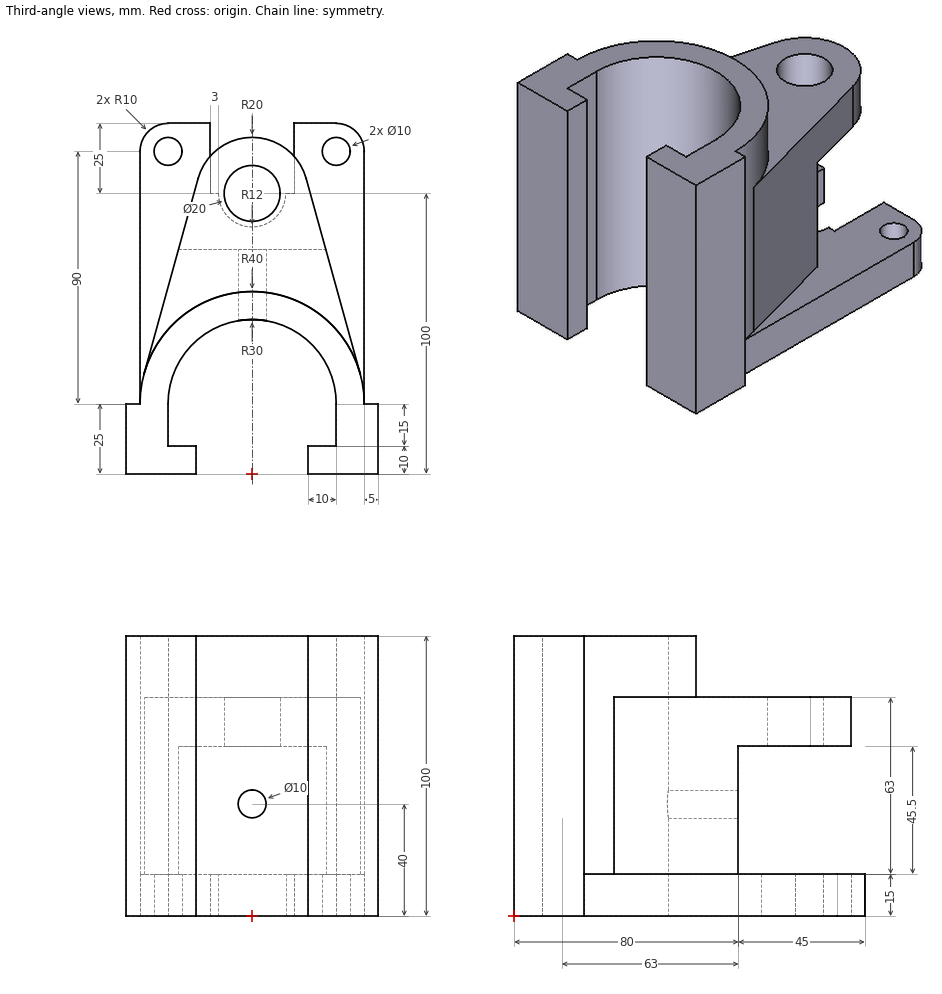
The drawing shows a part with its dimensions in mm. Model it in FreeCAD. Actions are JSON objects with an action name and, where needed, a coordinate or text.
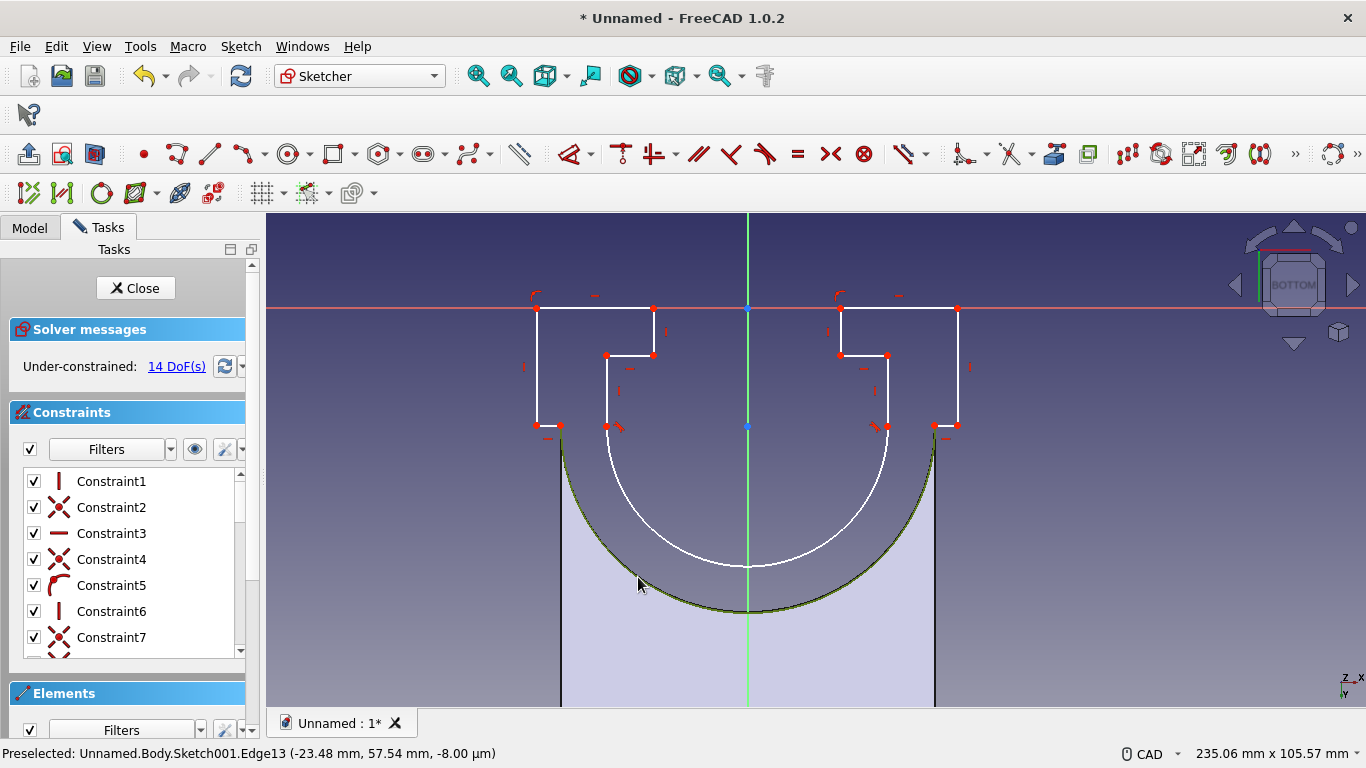
{"action": "left_click", "coordinate": [665, 540]}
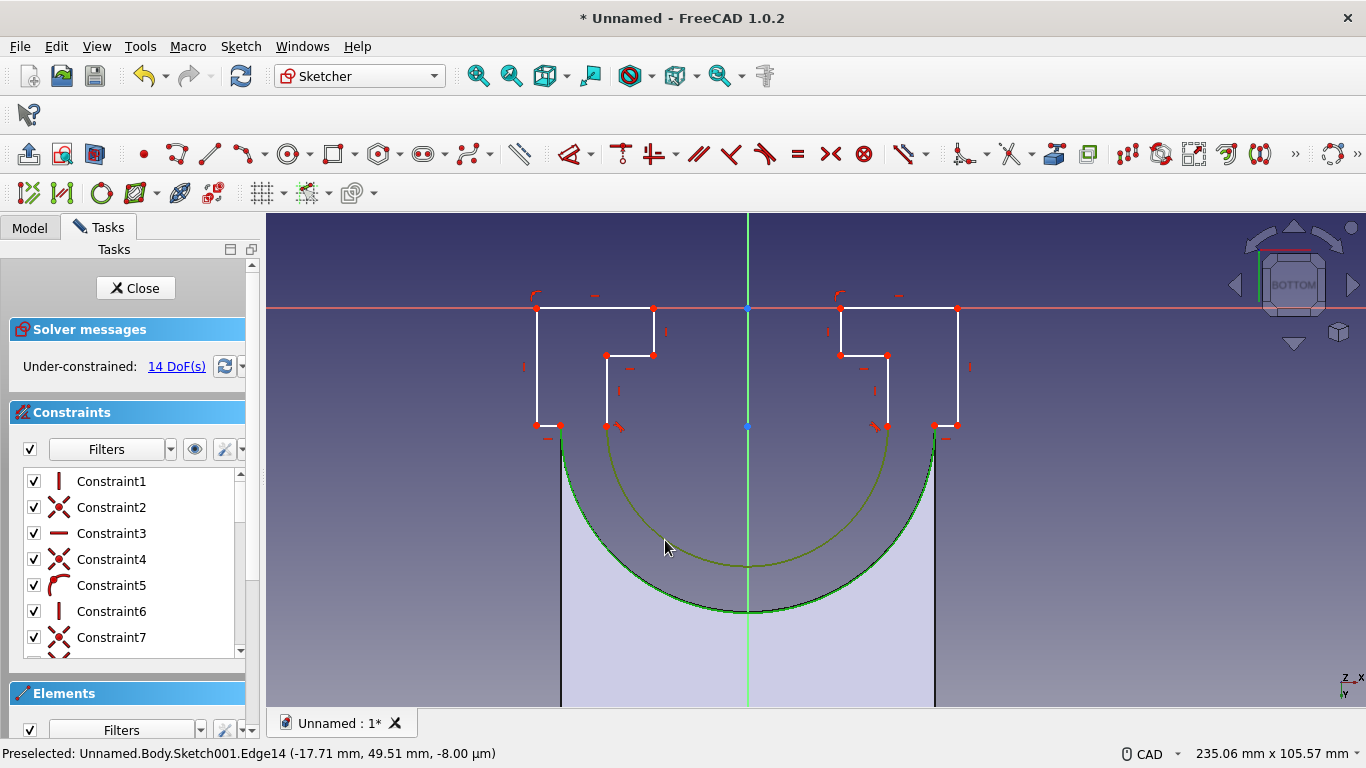
{"action": "key", "text": "c"}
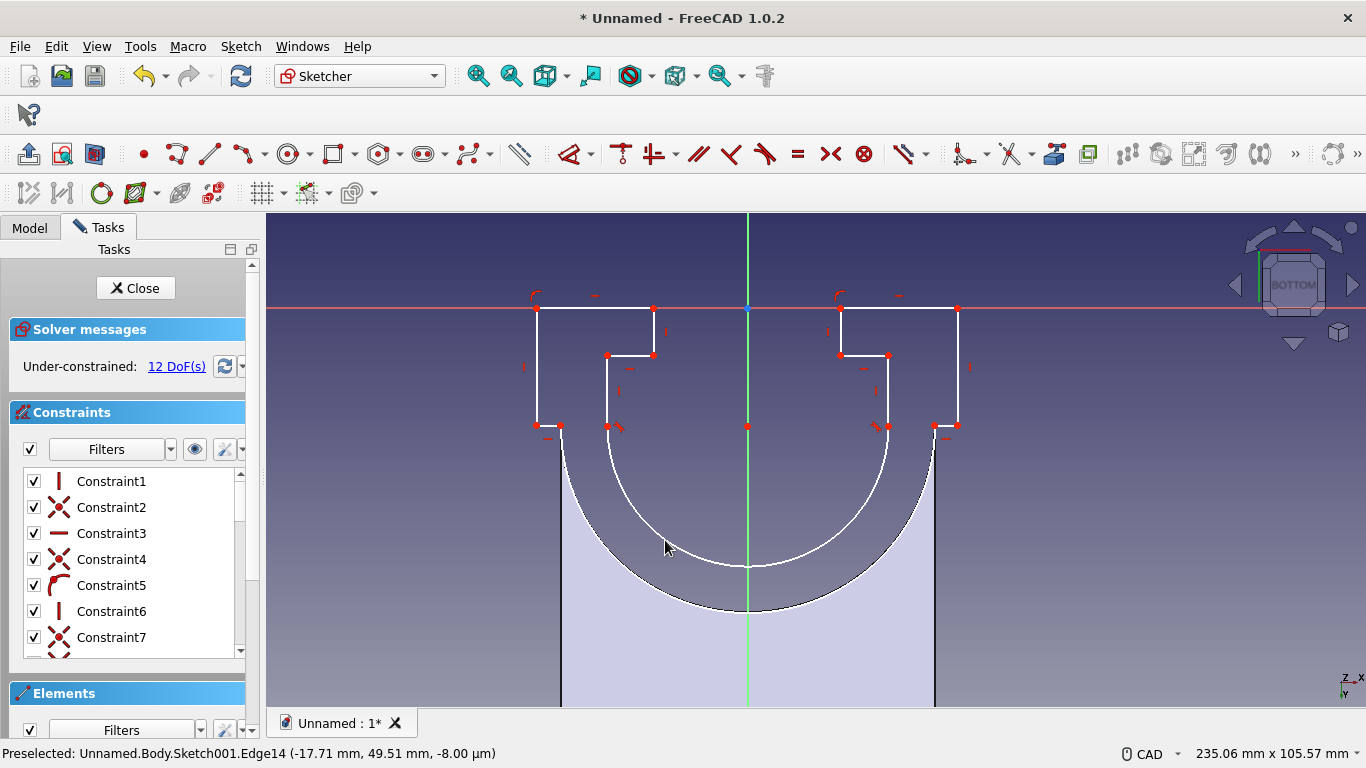
{"action": "left_click", "coordinate": [748, 426]}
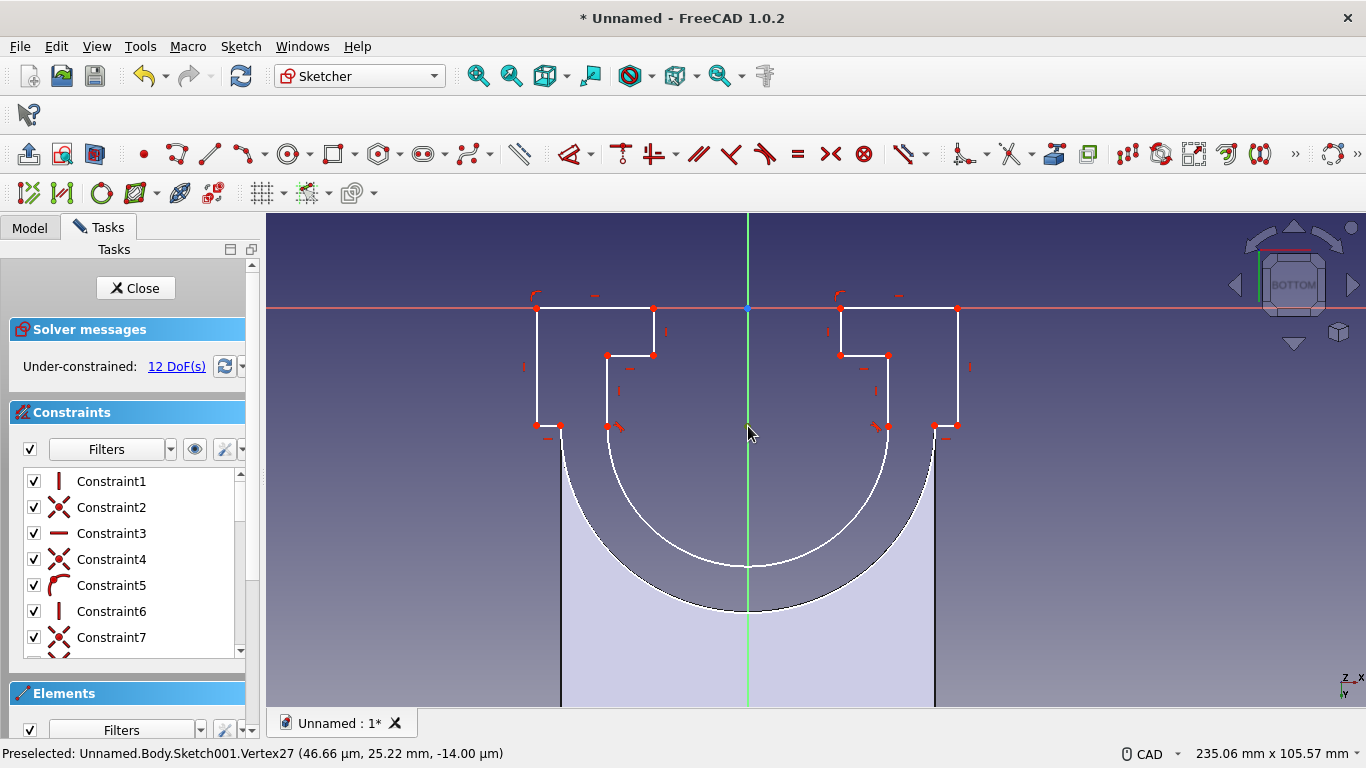
{"action": "left_click", "coordinate": [748, 648]}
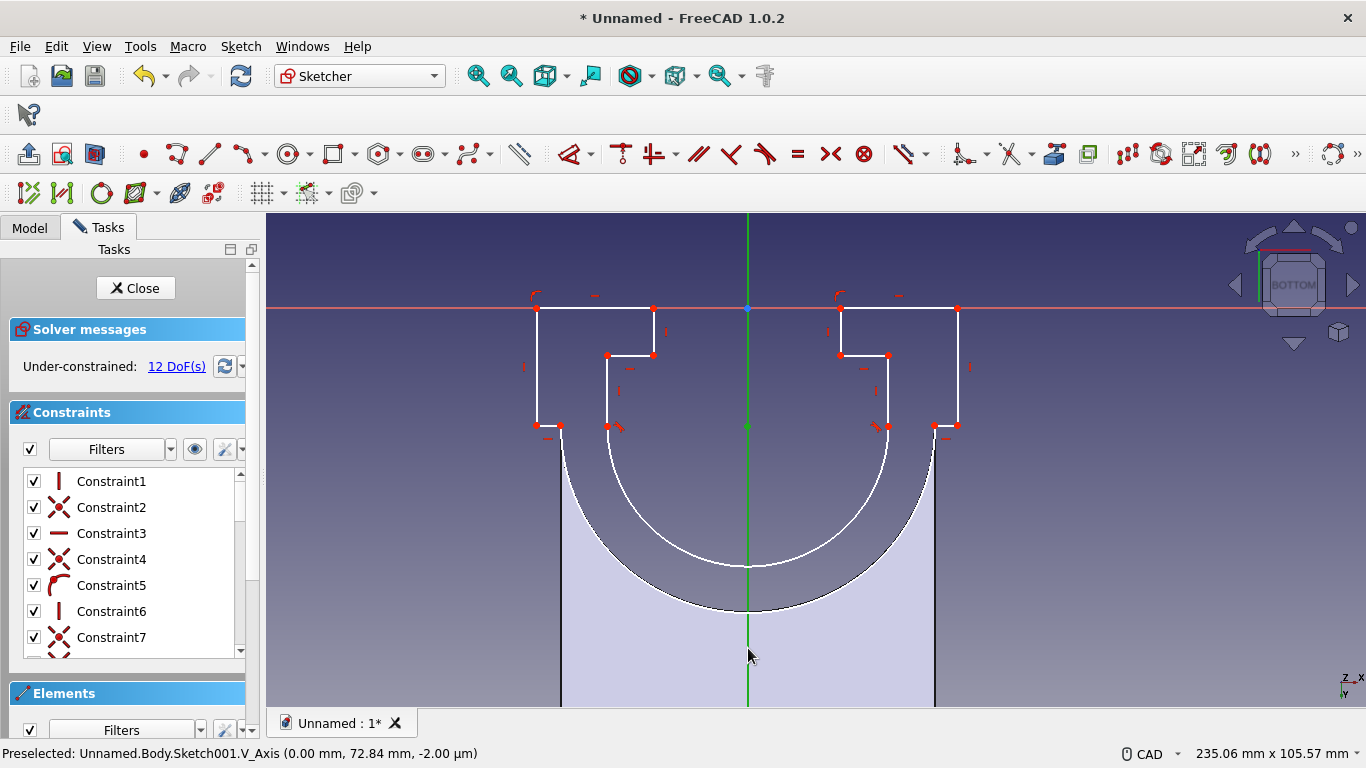
{"action": "key", "text": "c"}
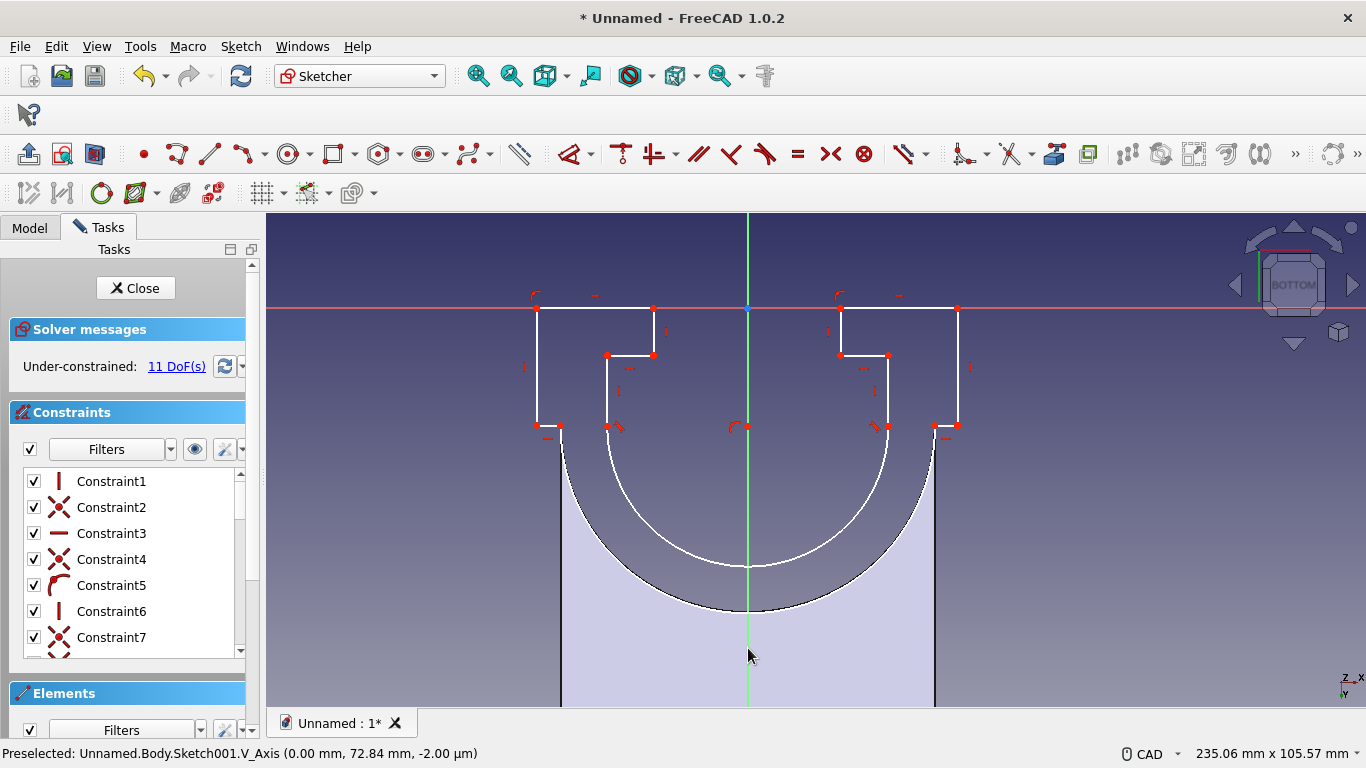
{"action": "left_click", "coordinate": [958, 426]}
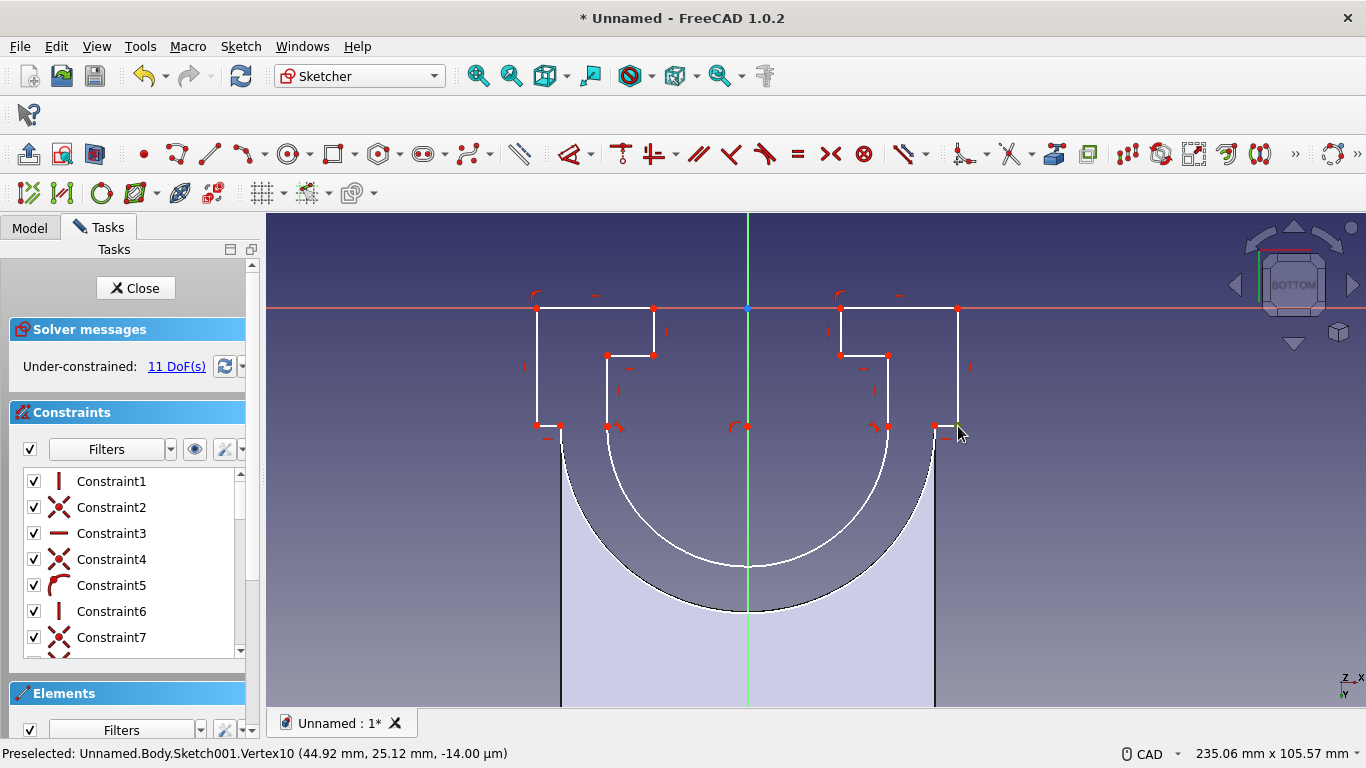
{"action": "left_click", "coordinate": [537, 426]}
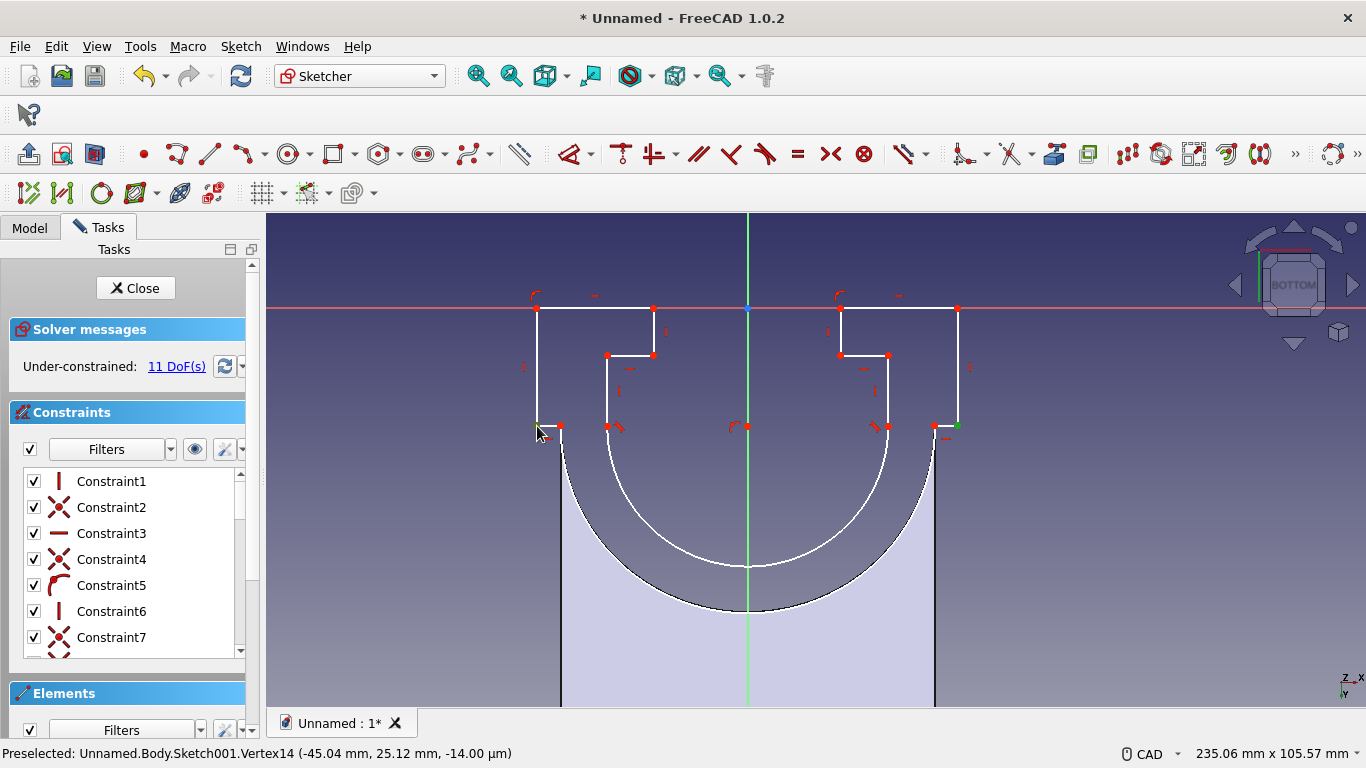
{"action": "left_click", "coordinate": [748, 648]}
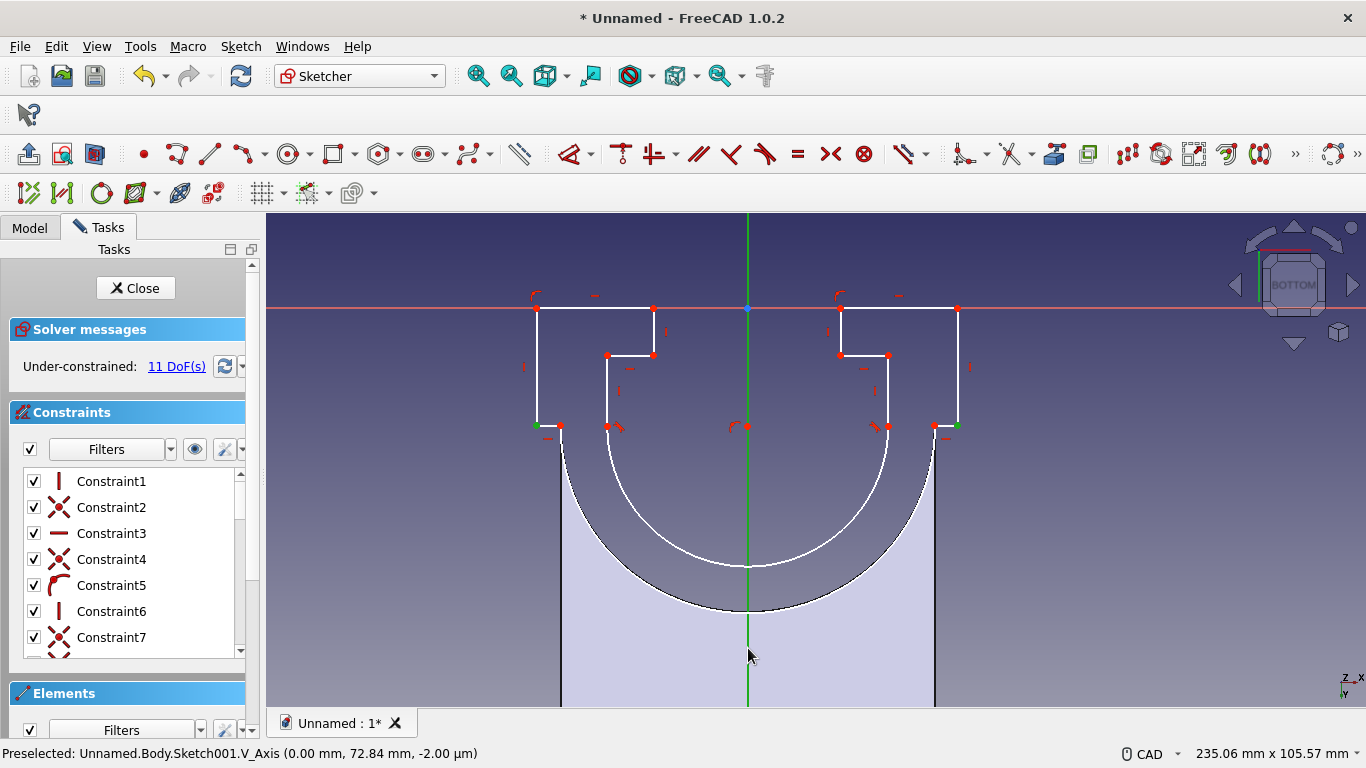
{"action": "key", "text": "s"}